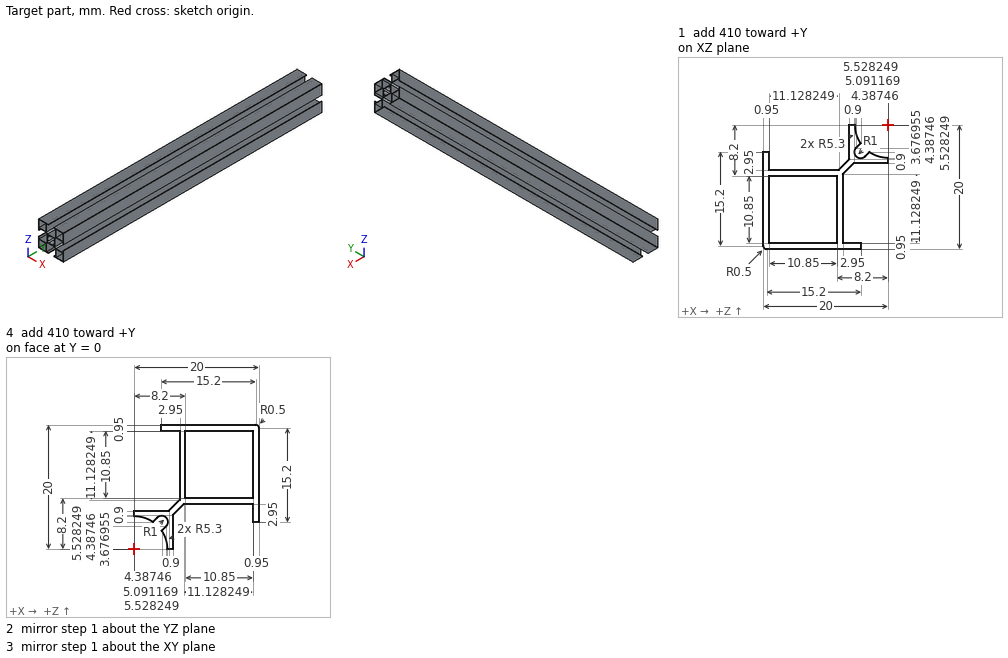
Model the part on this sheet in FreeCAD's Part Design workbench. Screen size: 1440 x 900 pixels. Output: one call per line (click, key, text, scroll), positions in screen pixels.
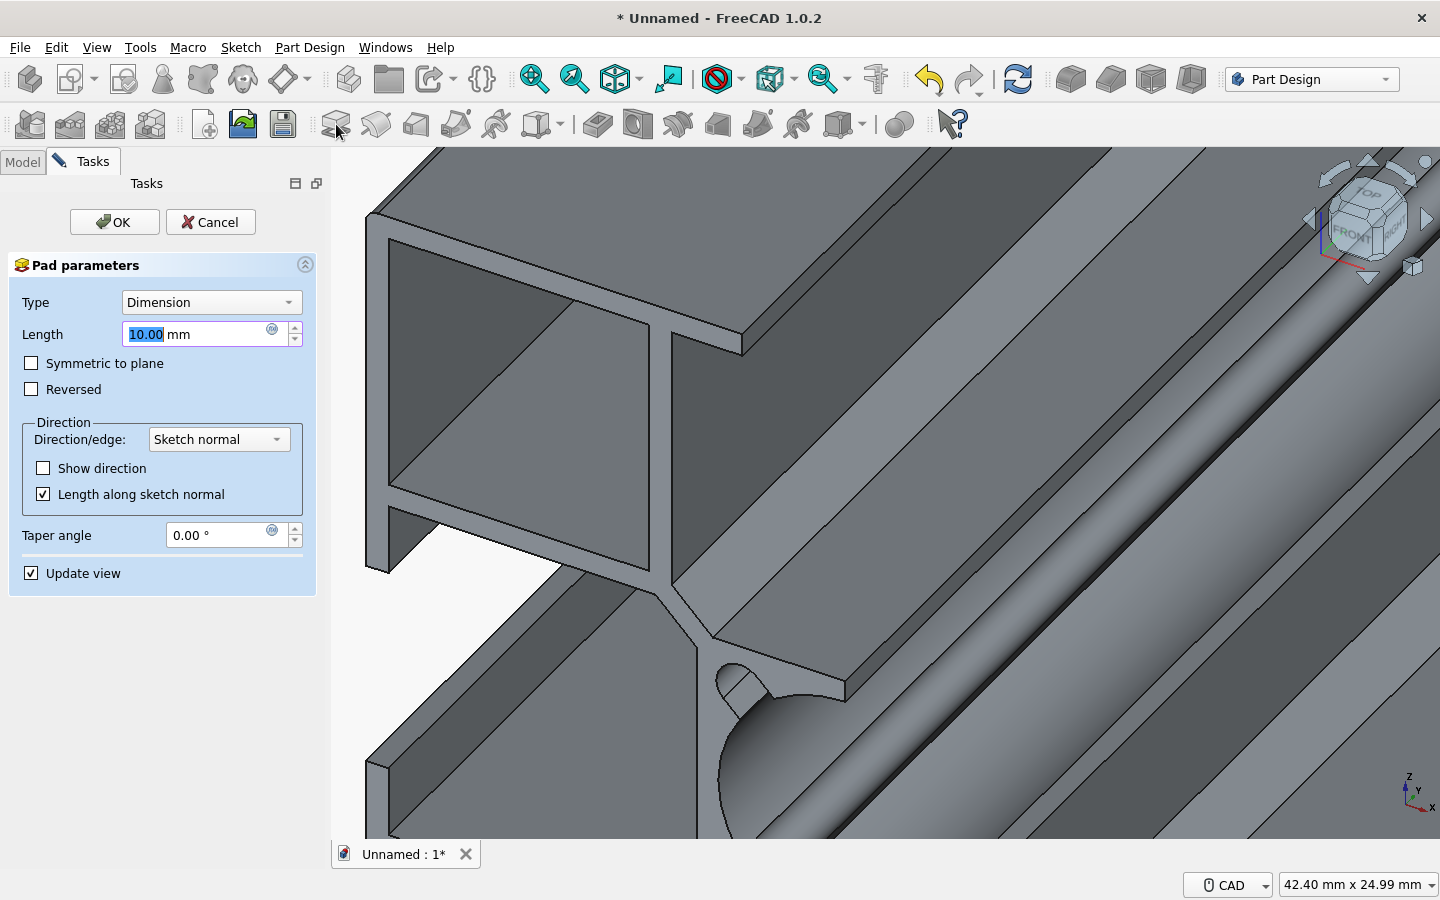
text(410)
key(Tab)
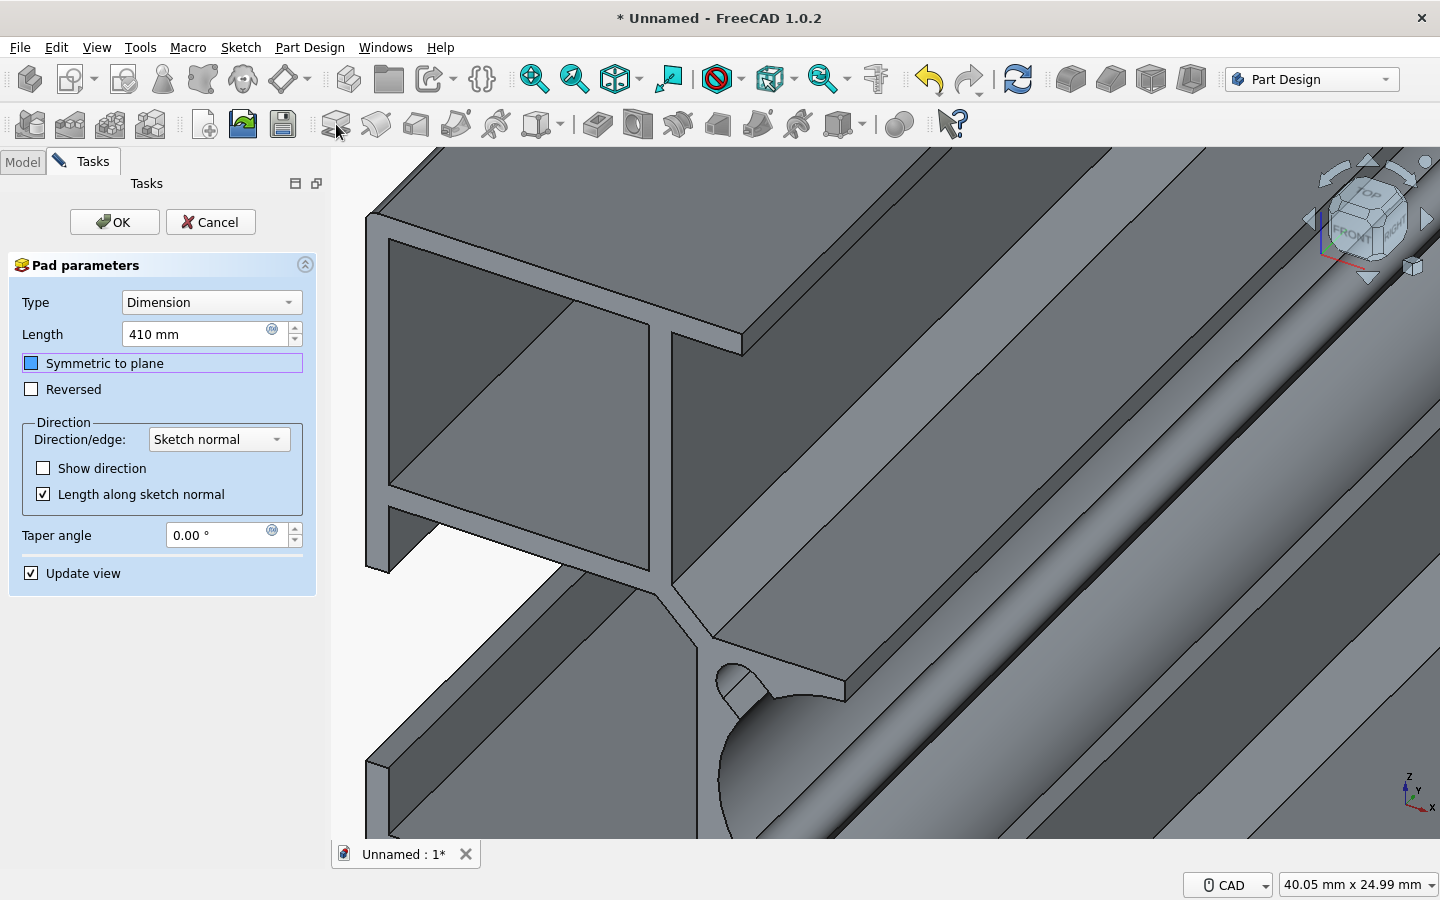
click(30, 389)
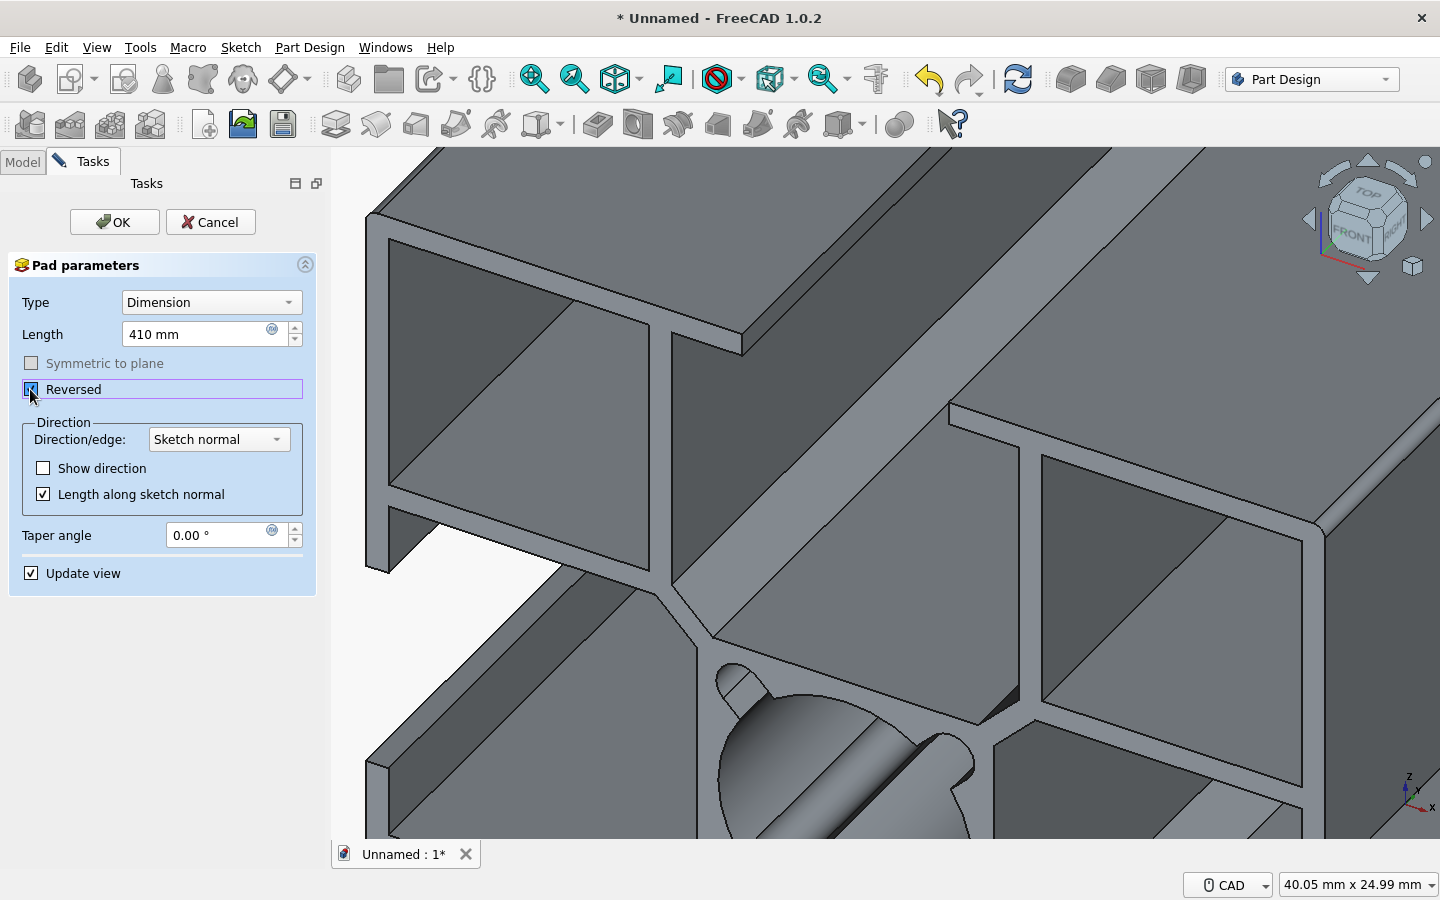
click(115, 222)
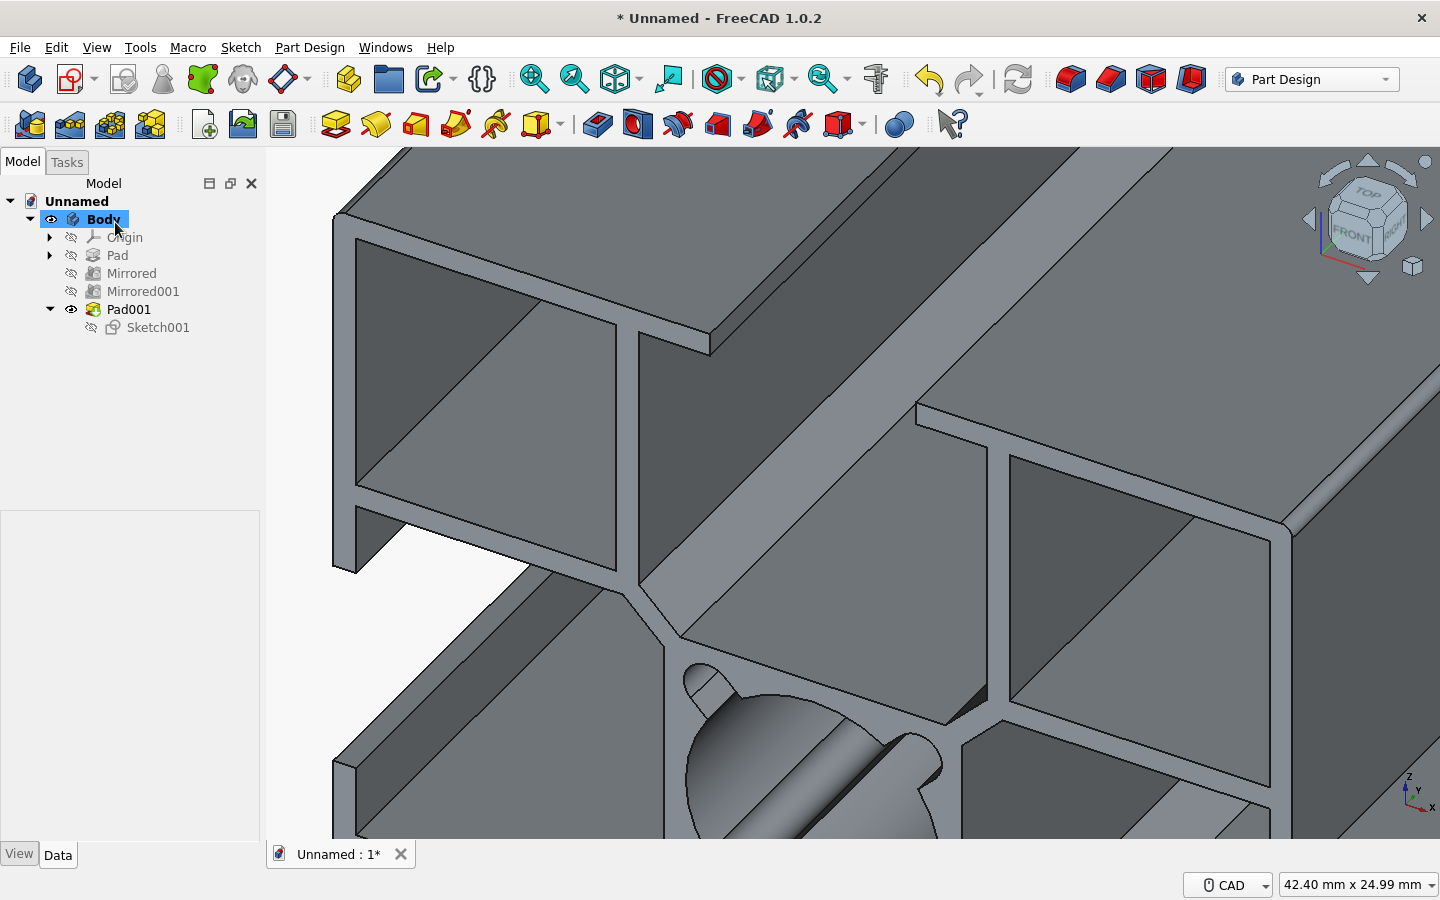
key(0)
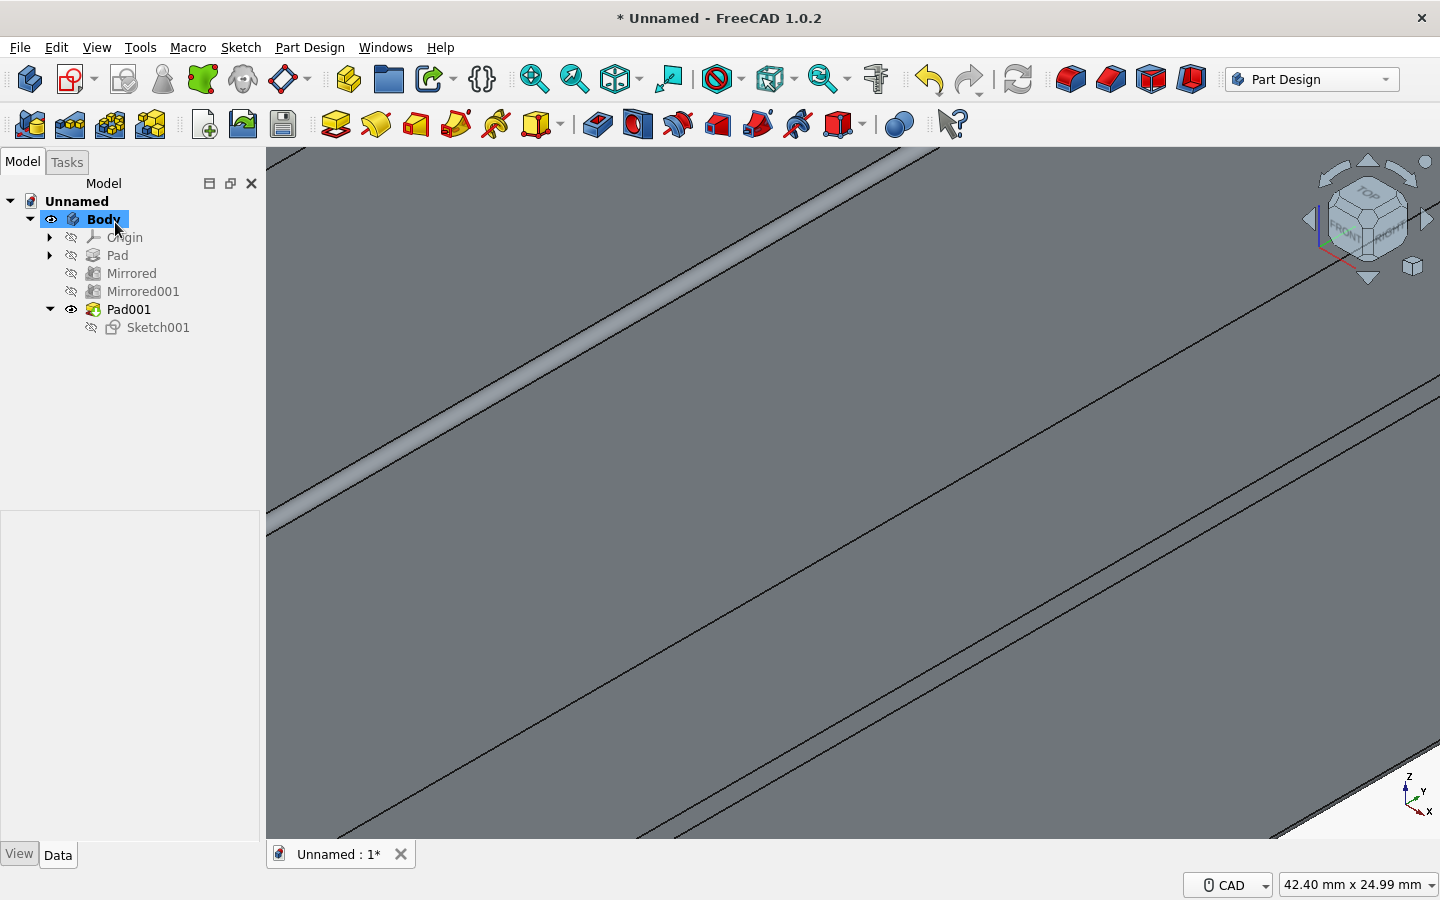
click(536, 80)